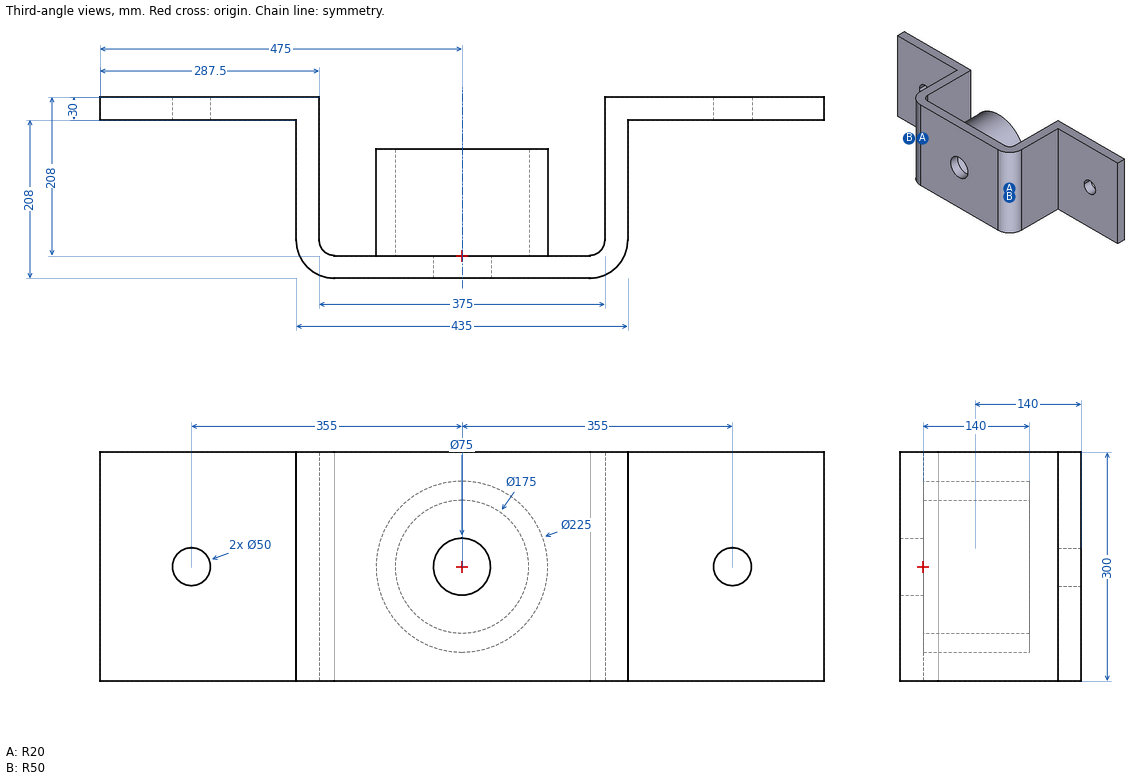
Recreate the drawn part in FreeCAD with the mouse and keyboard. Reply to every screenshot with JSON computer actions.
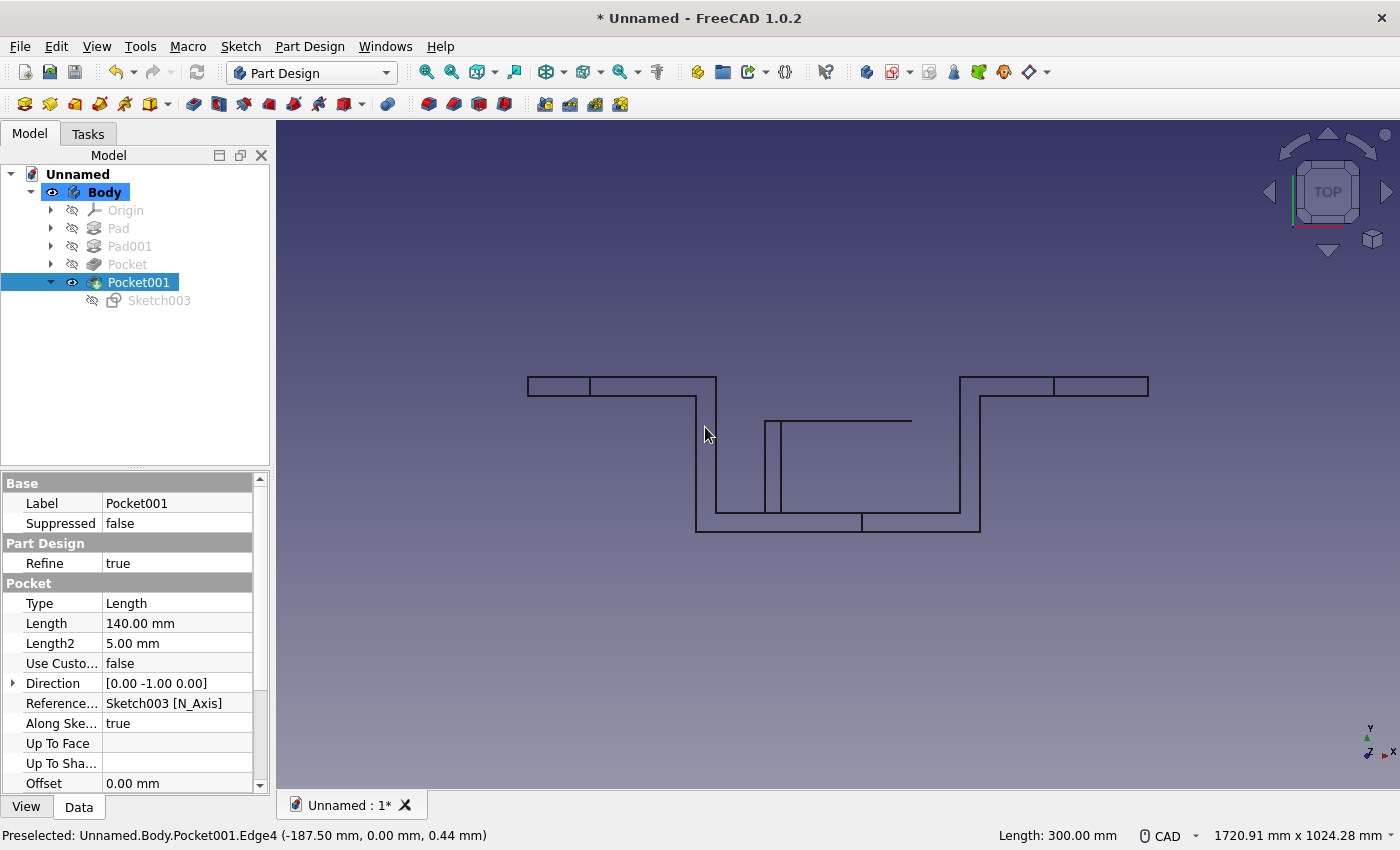
{"action": "key", "text": "1"}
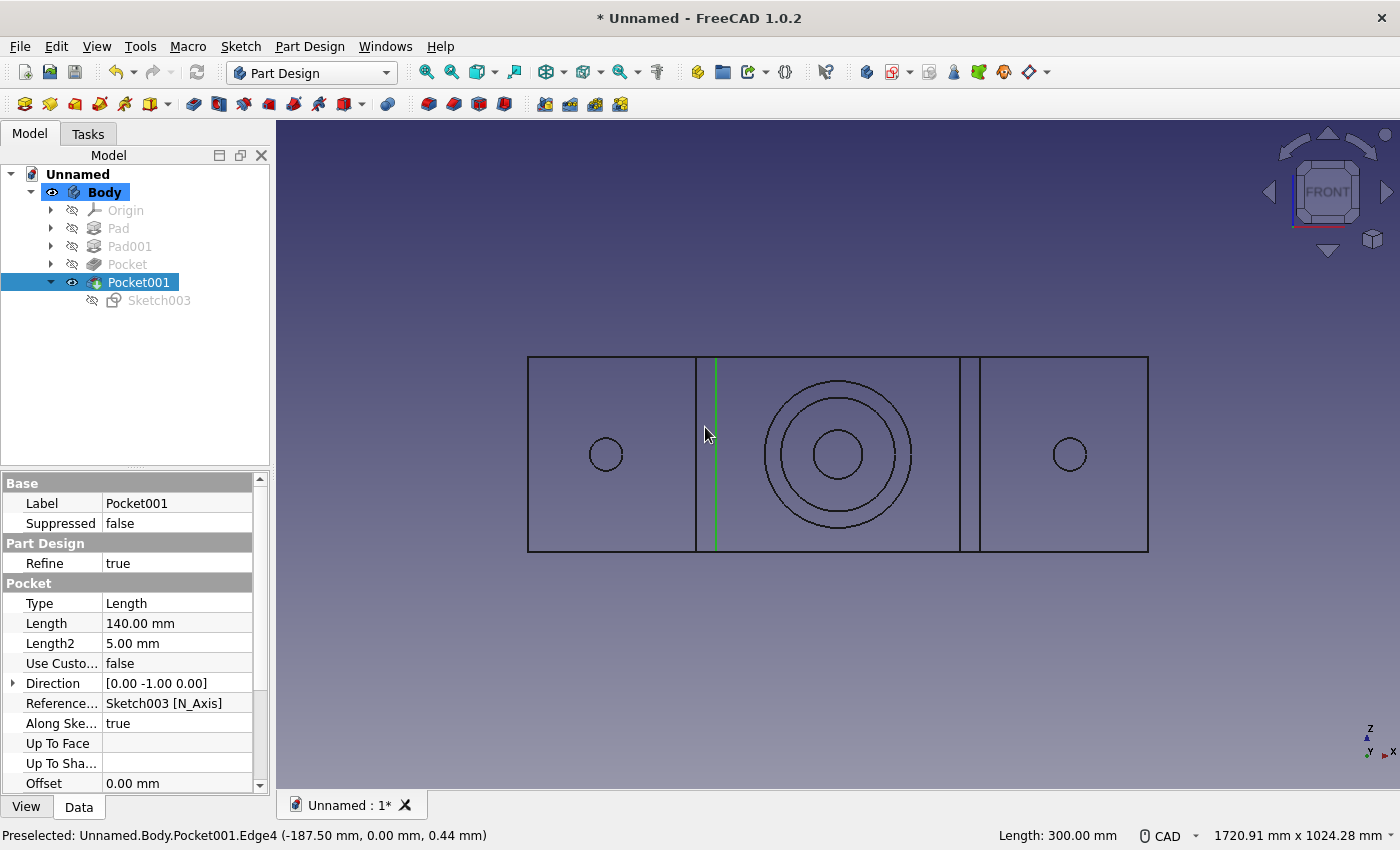
{"action": "left_click", "coordinate": [960, 453], "text": "ctrl"}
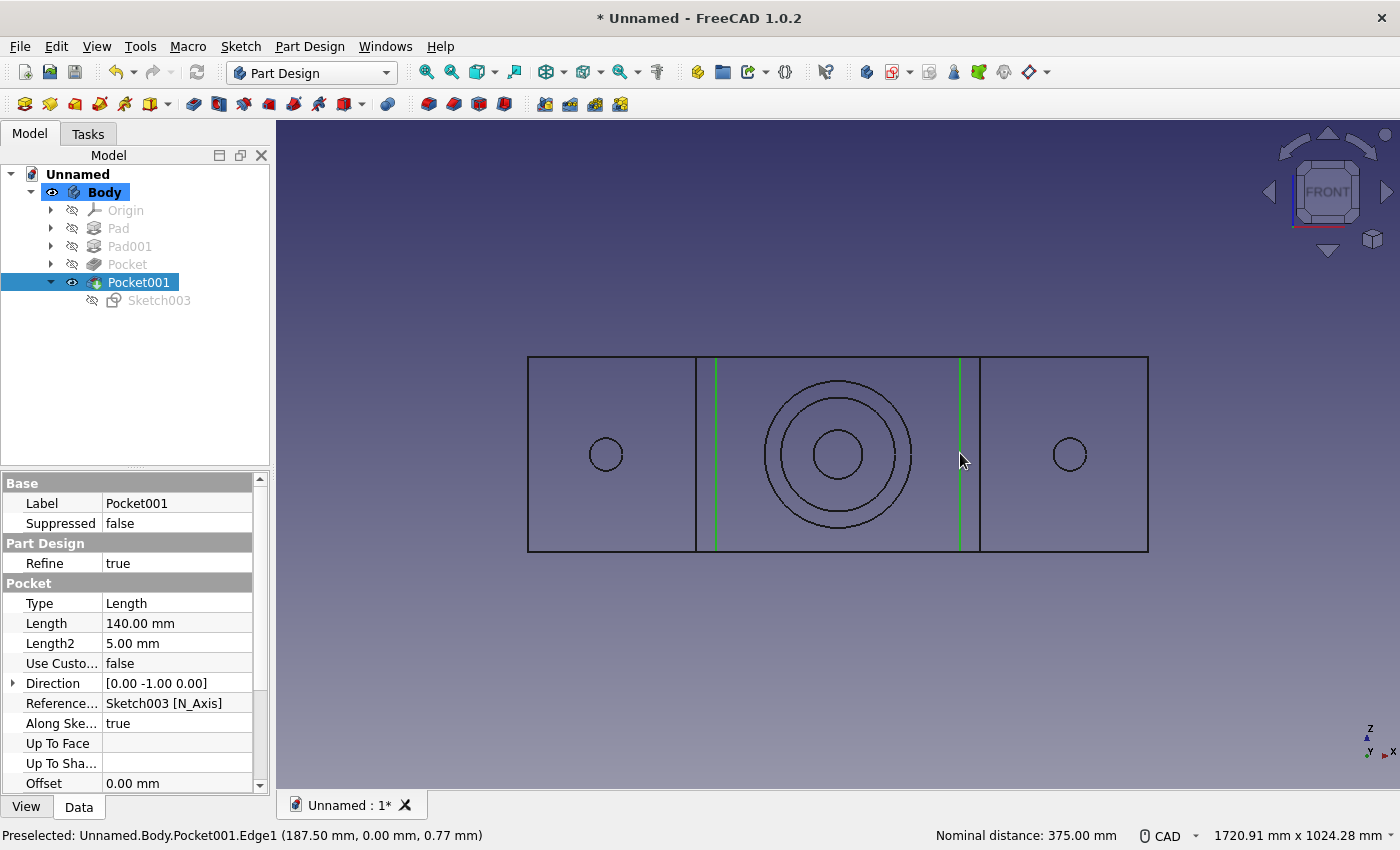
{"action": "key", "text": "v 1"}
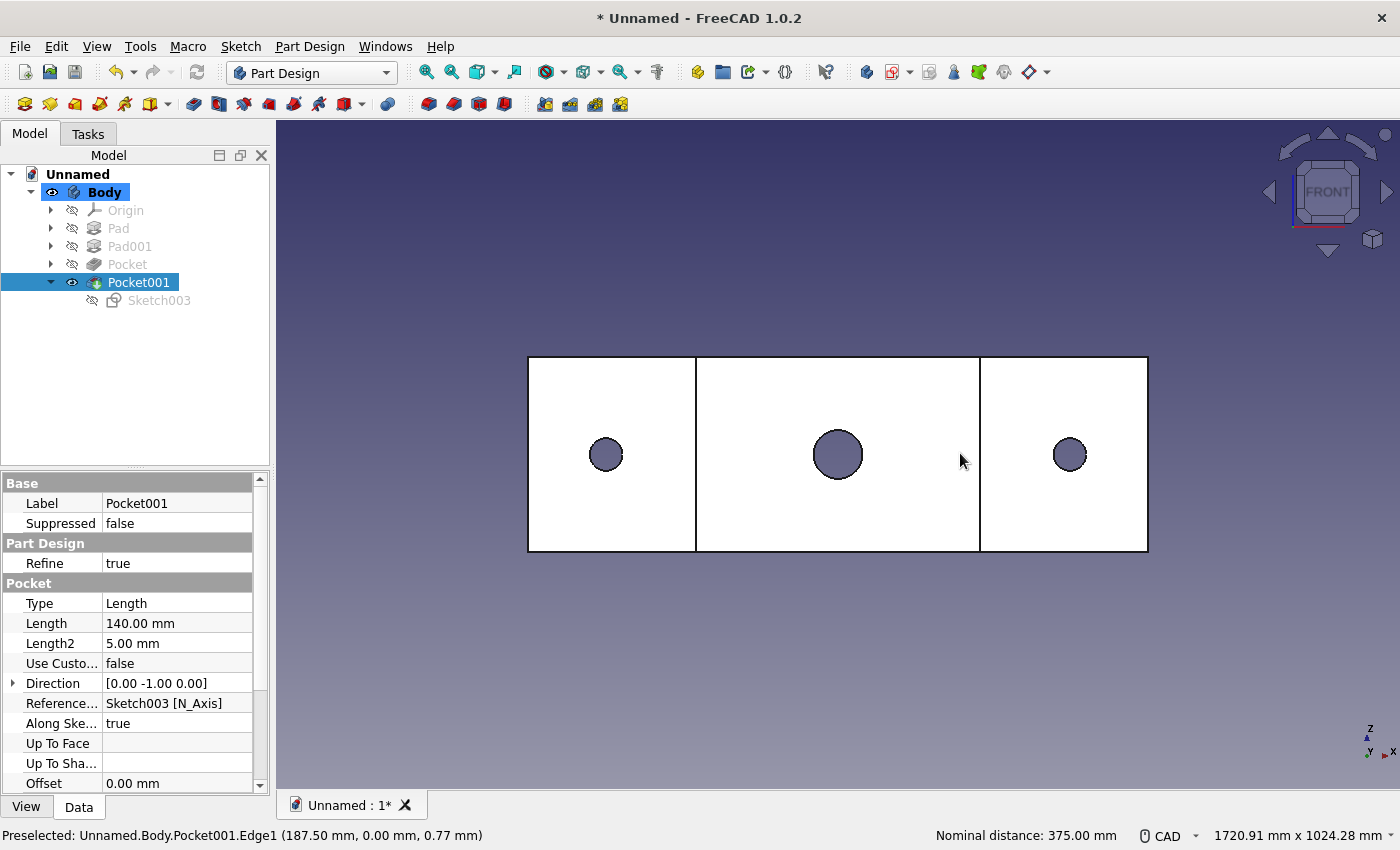
{"action": "left_click", "coordinate": [429, 104]}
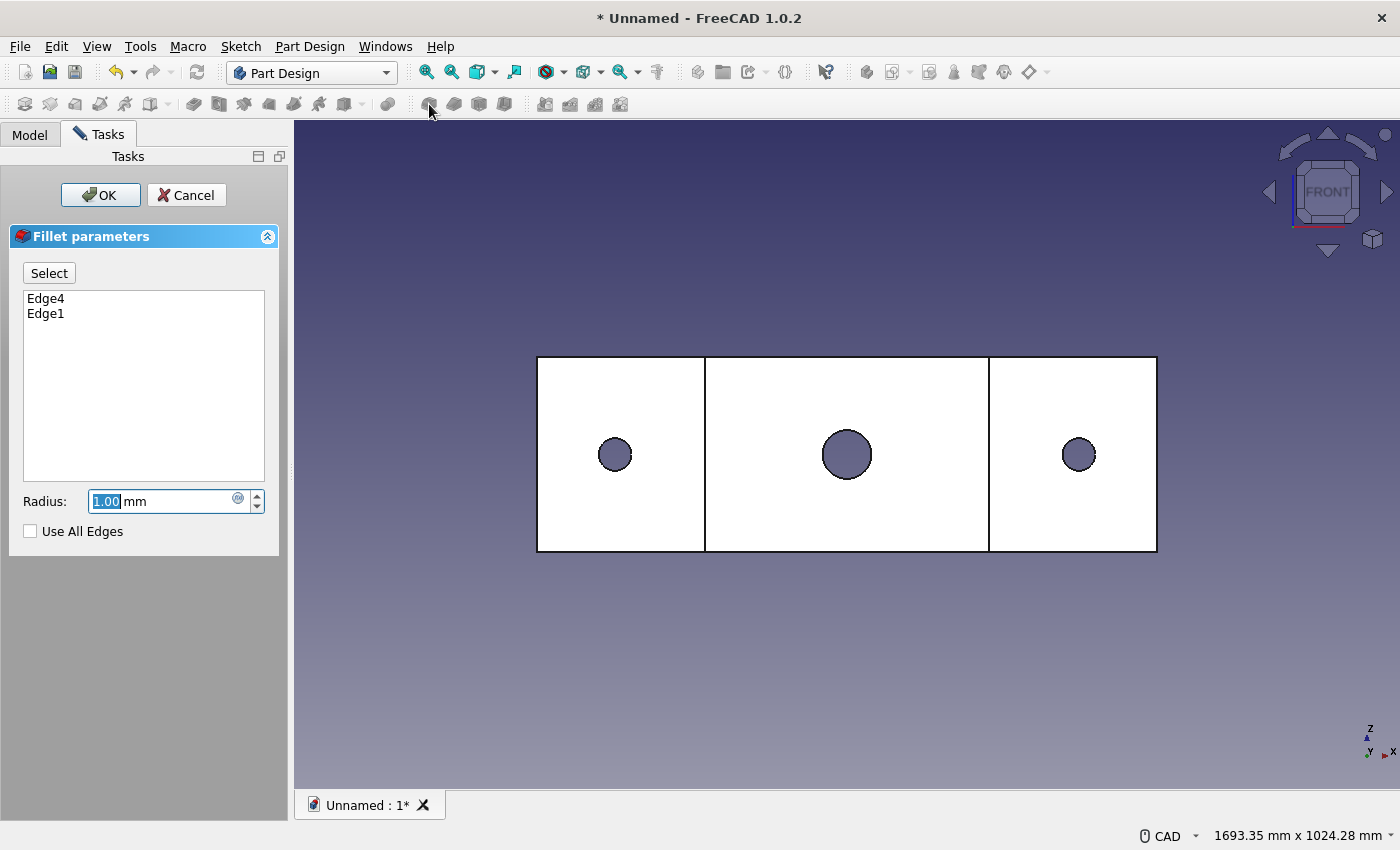
{"action": "type", "text": "20"}
{"action": "key", "text": "Tab"}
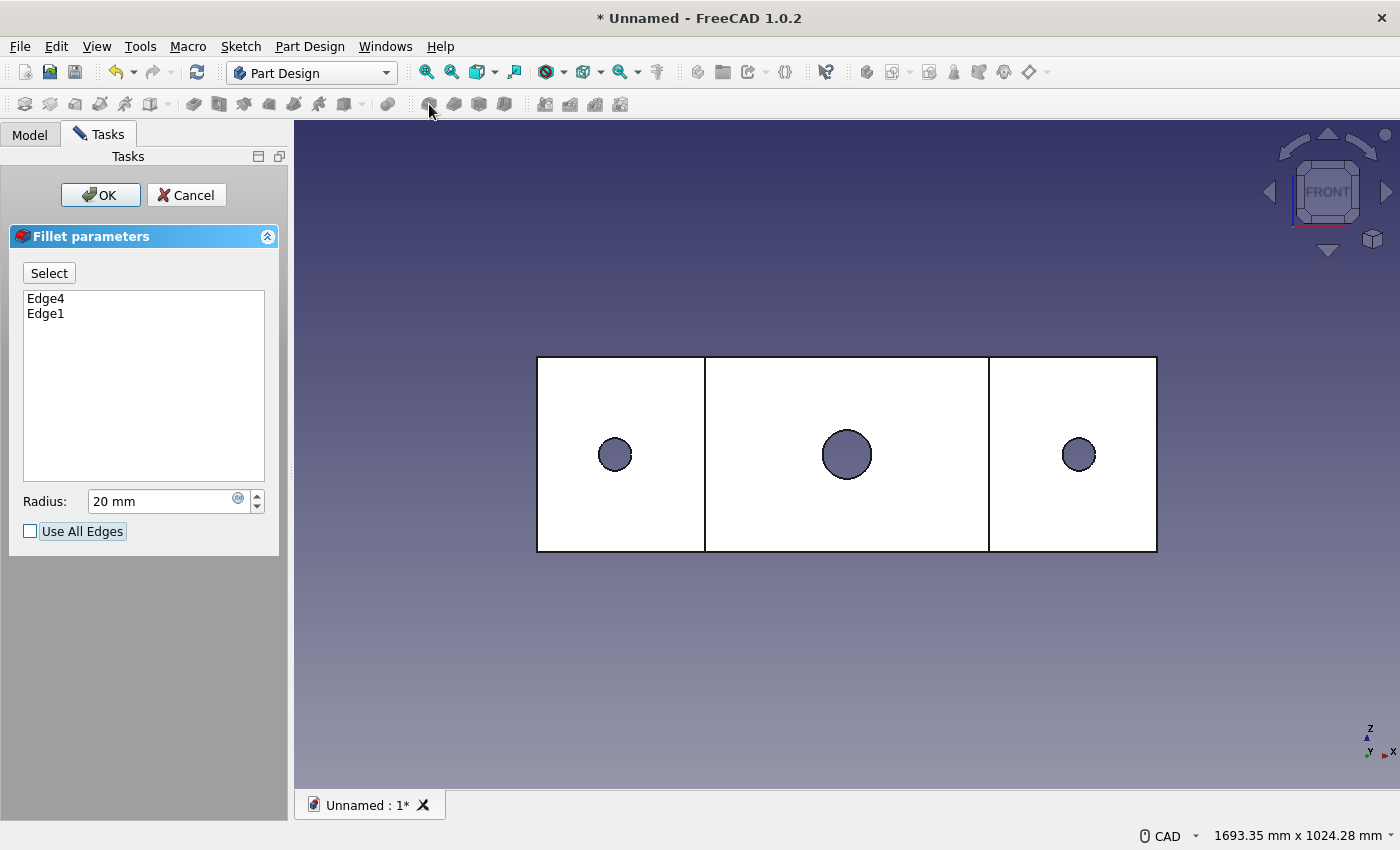
{"action": "left_click", "coordinate": [101, 195]}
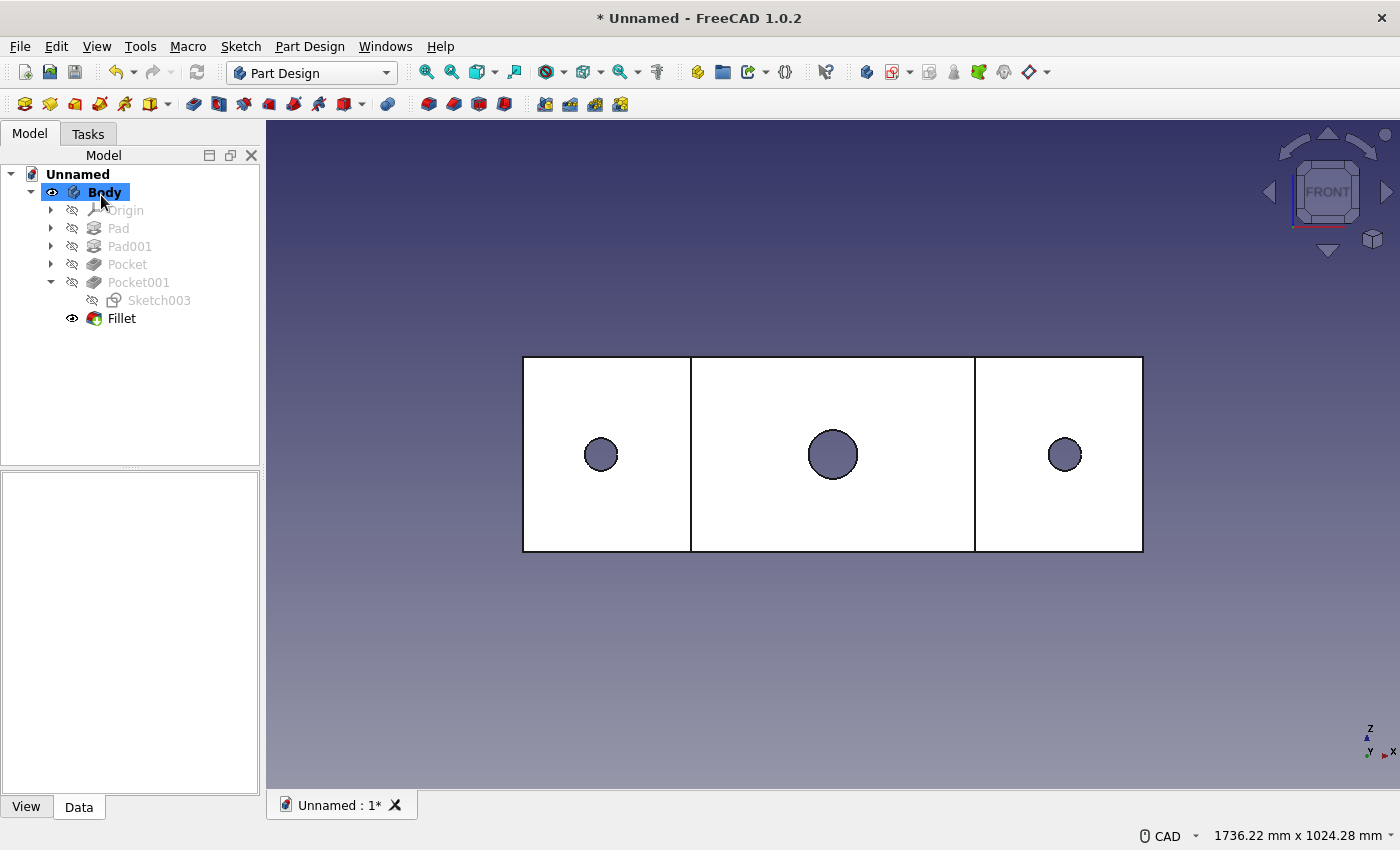
{"action": "left_click", "coordinate": [975, 453]}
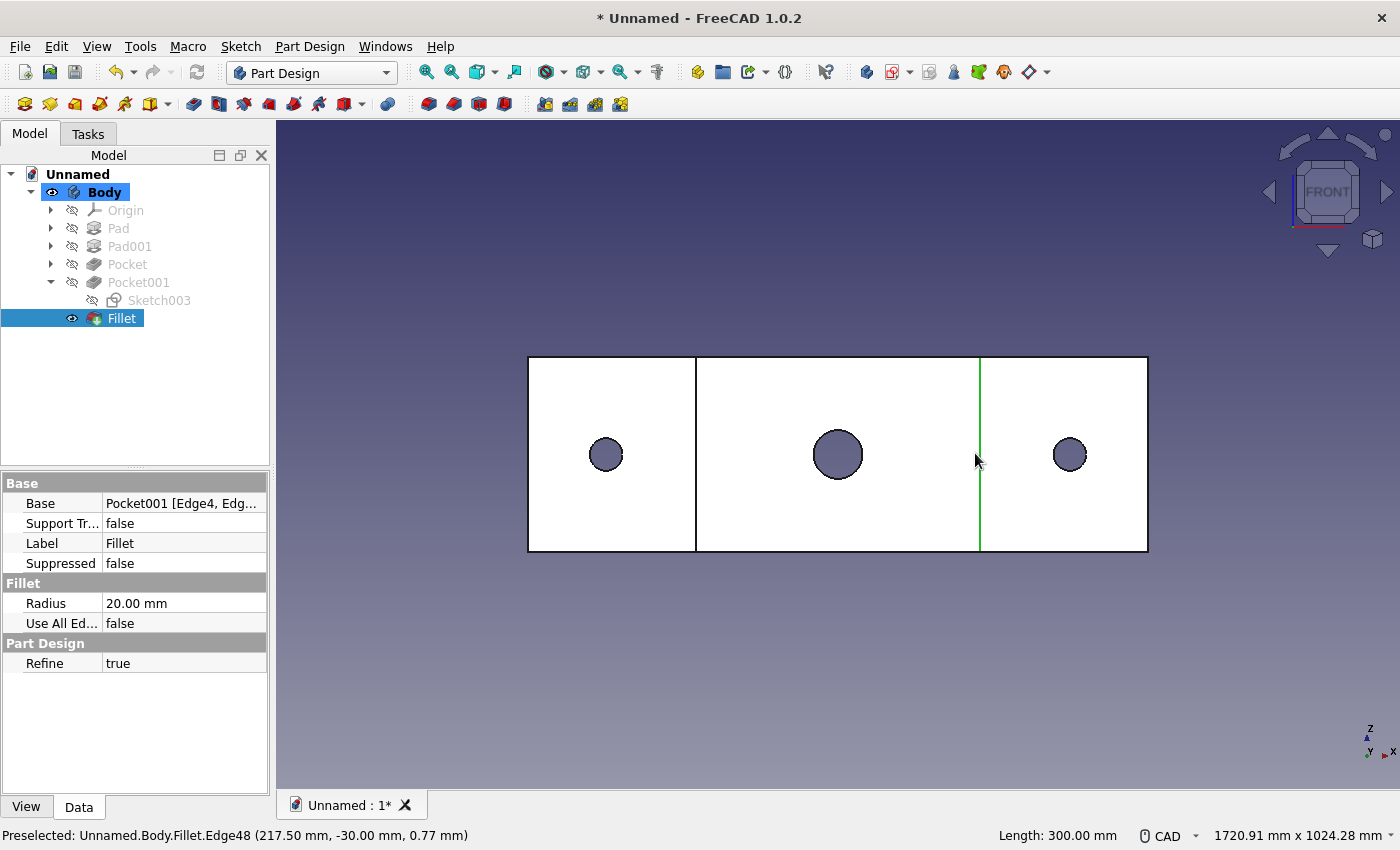
{"action": "left_click", "coordinate": [696, 453], "text": "ctrl"}